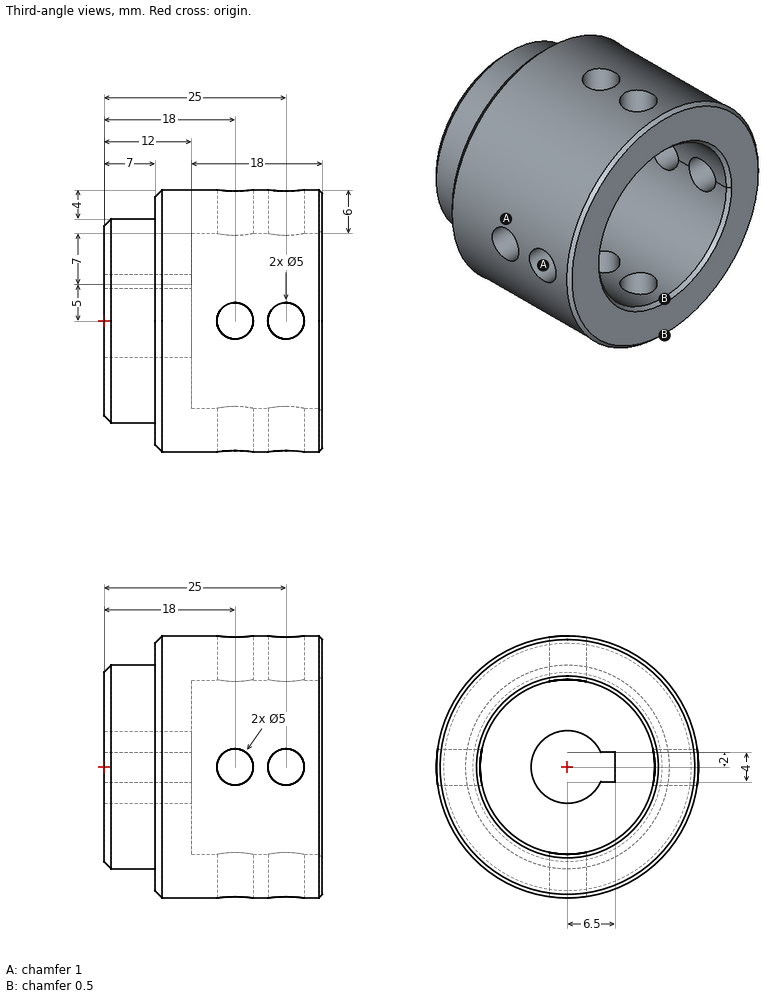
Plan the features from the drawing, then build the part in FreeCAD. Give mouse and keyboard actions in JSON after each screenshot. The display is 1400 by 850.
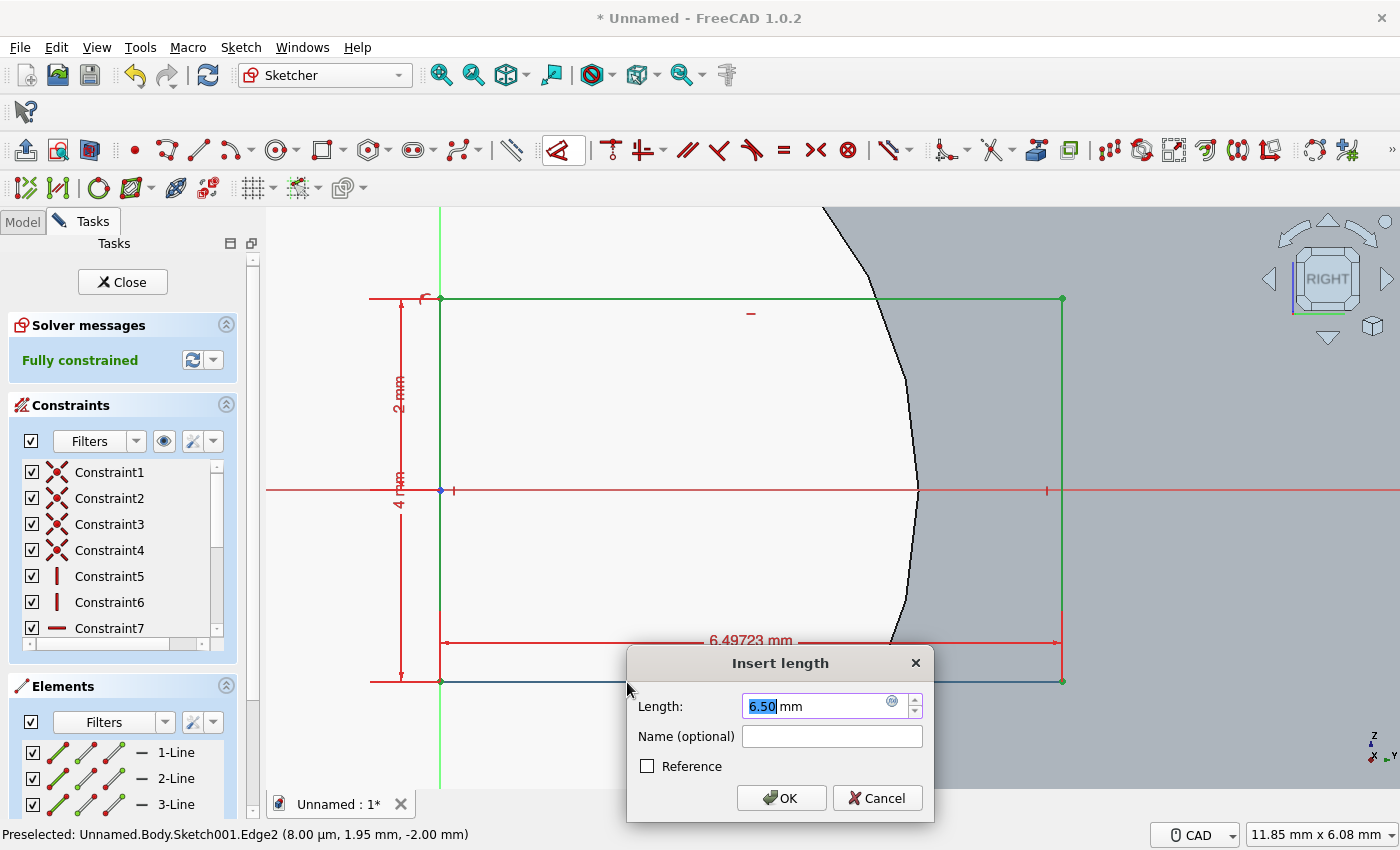
{"action": "type", "text": "6.5"}
{"action": "key", "text": "Return"}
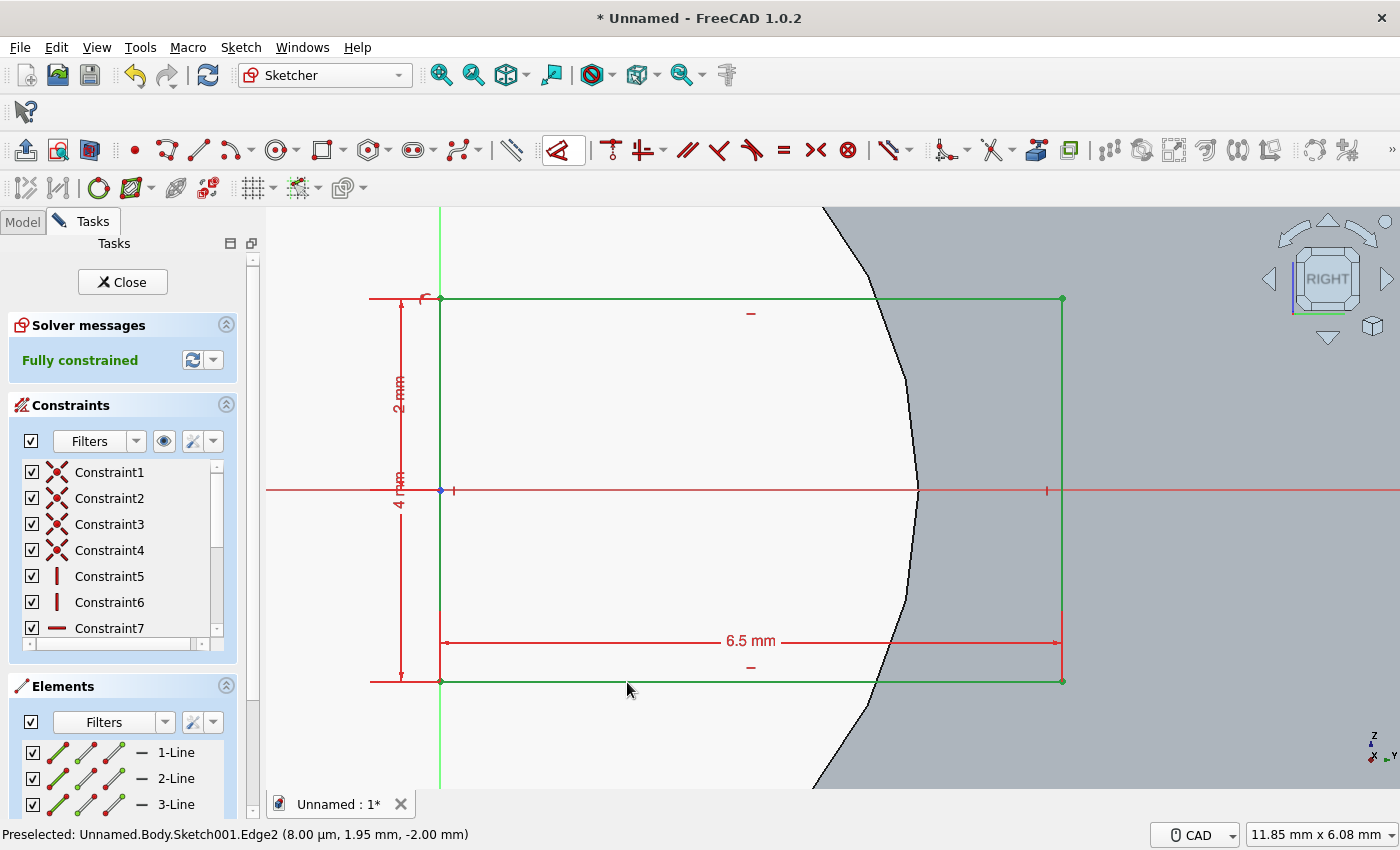
{"action": "left_click", "coordinate": [123, 282]}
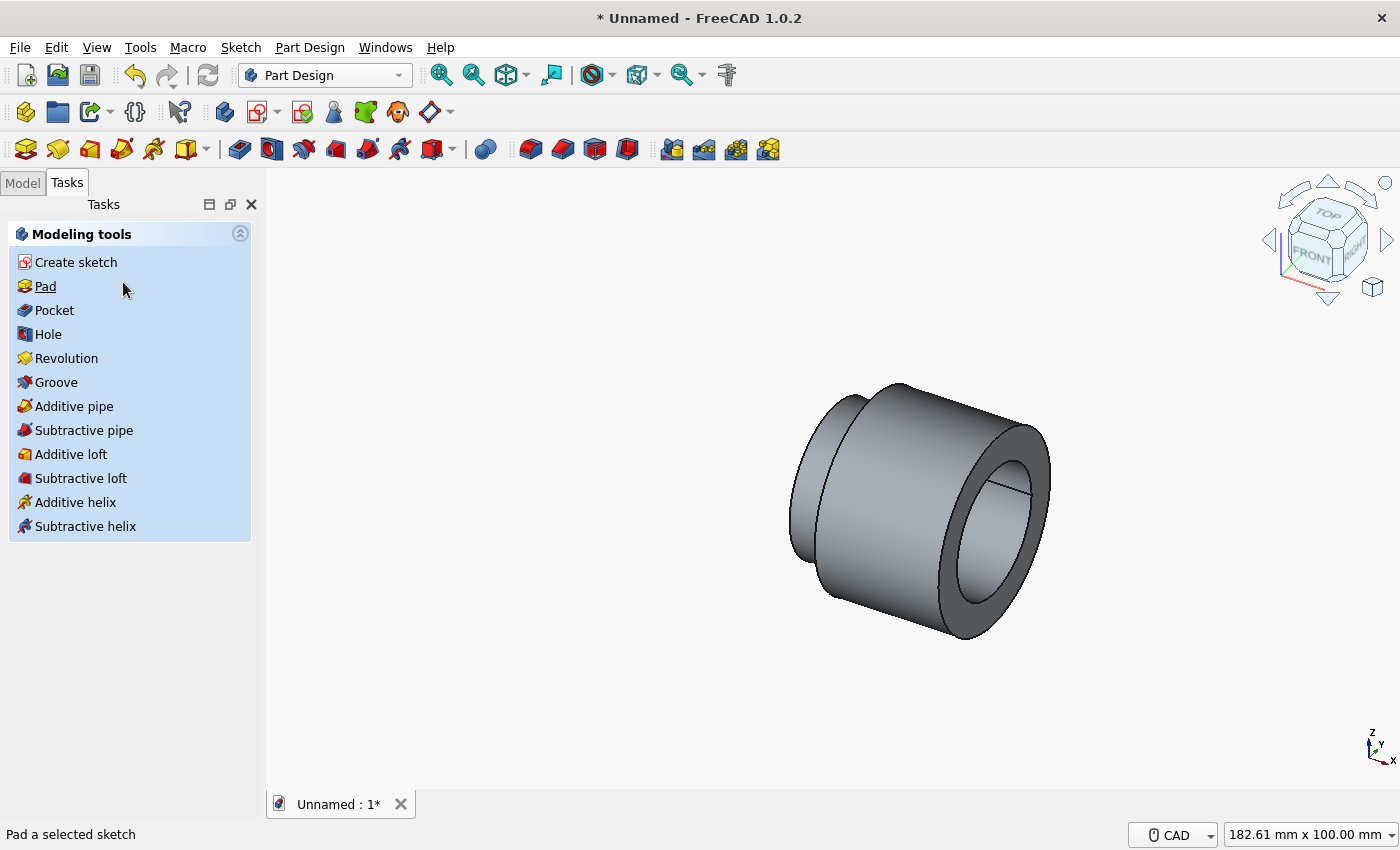
{"action": "left_click", "coordinate": [240, 150]}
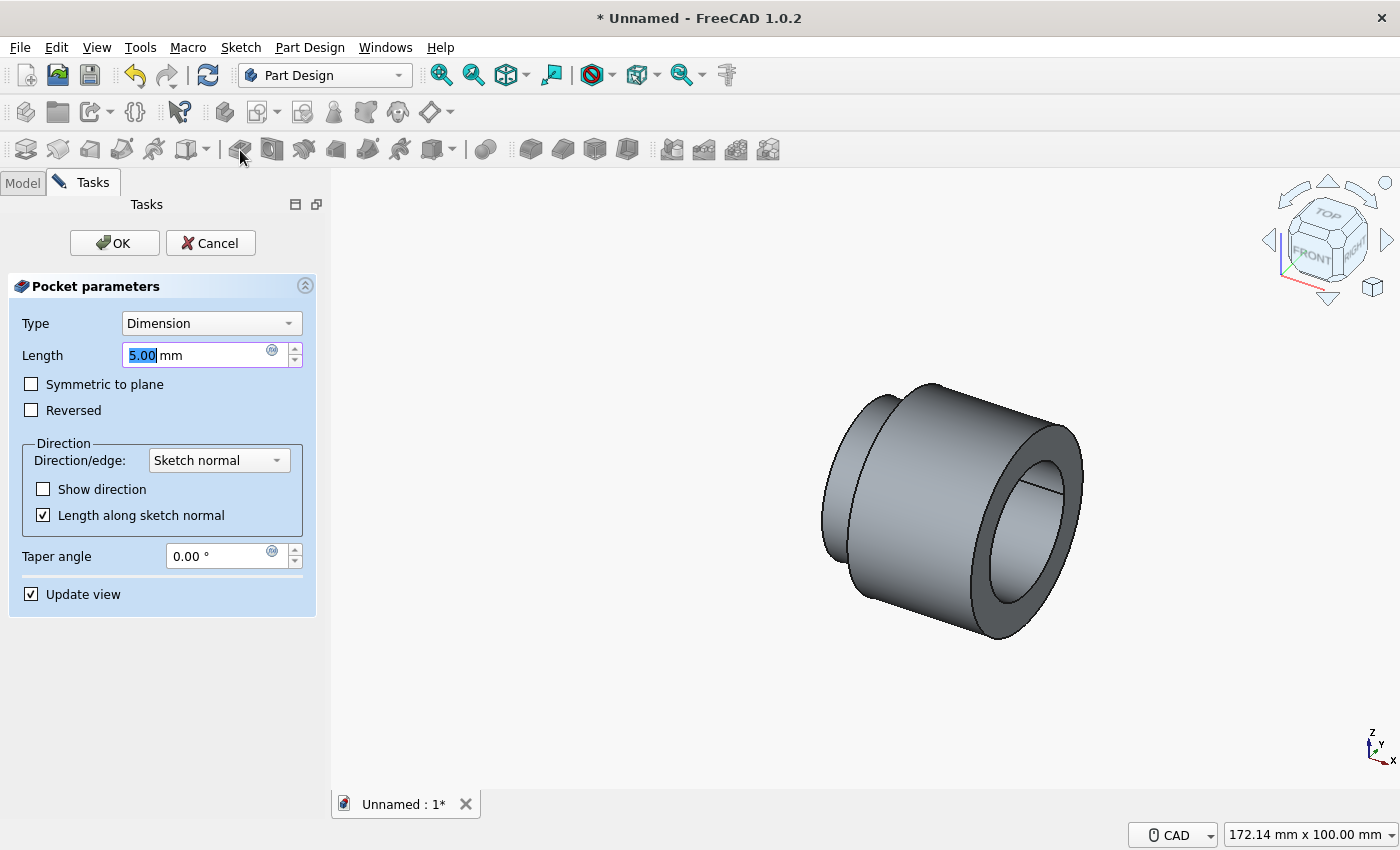
{"action": "left_click", "coordinate": [212, 324]}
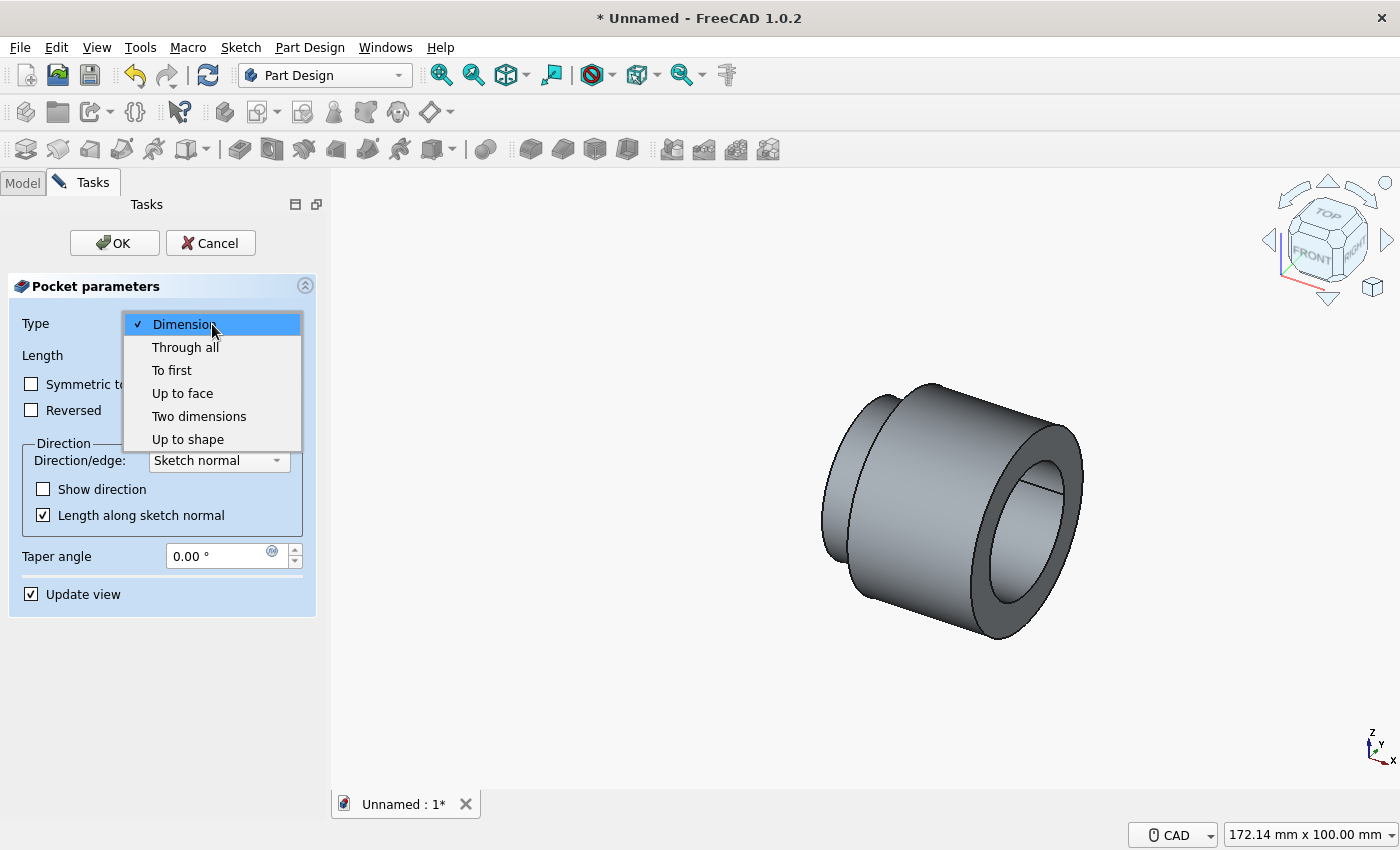
{"action": "left_click", "coordinate": [212, 348]}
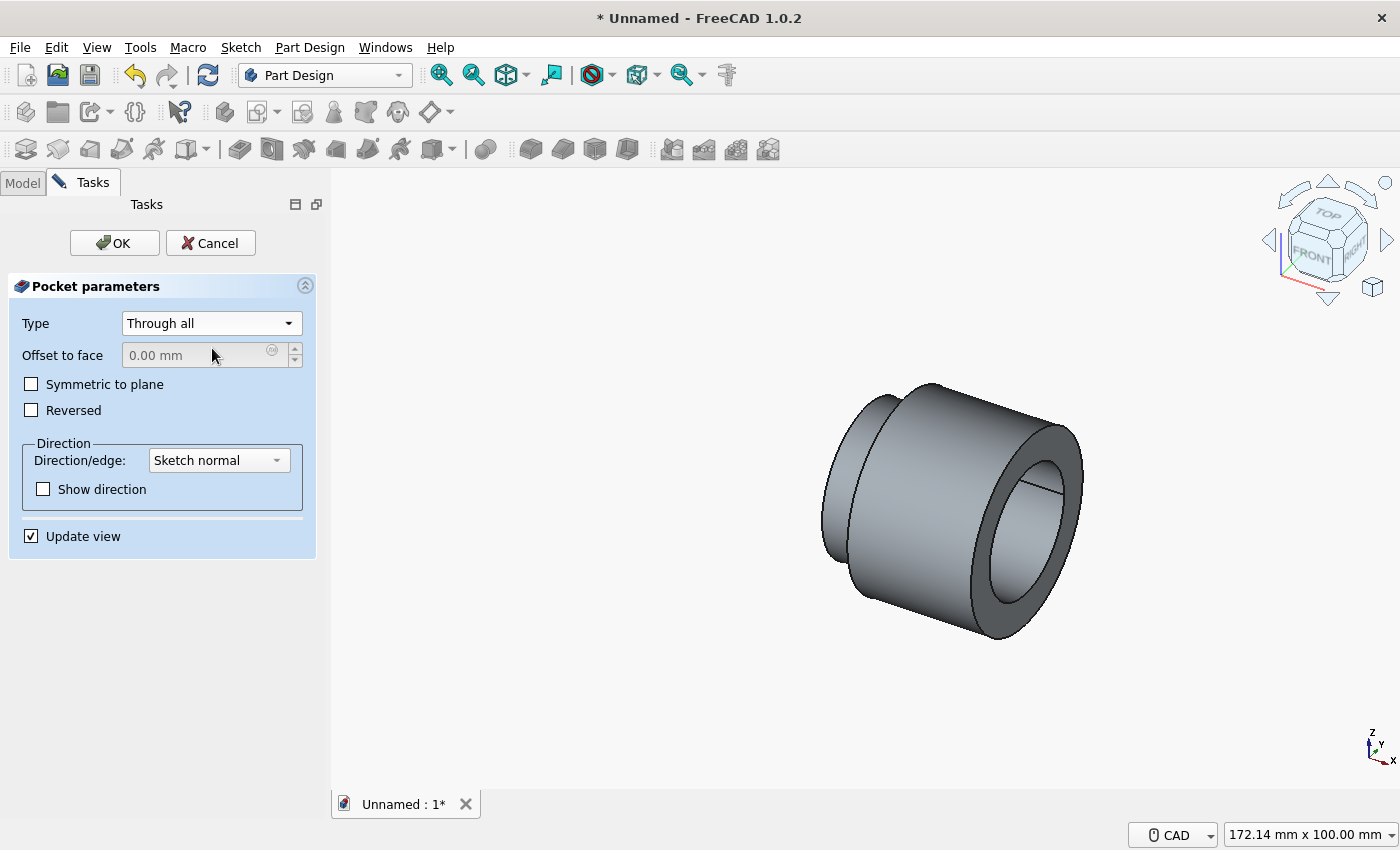
{"action": "left_click", "coordinate": [30, 410]}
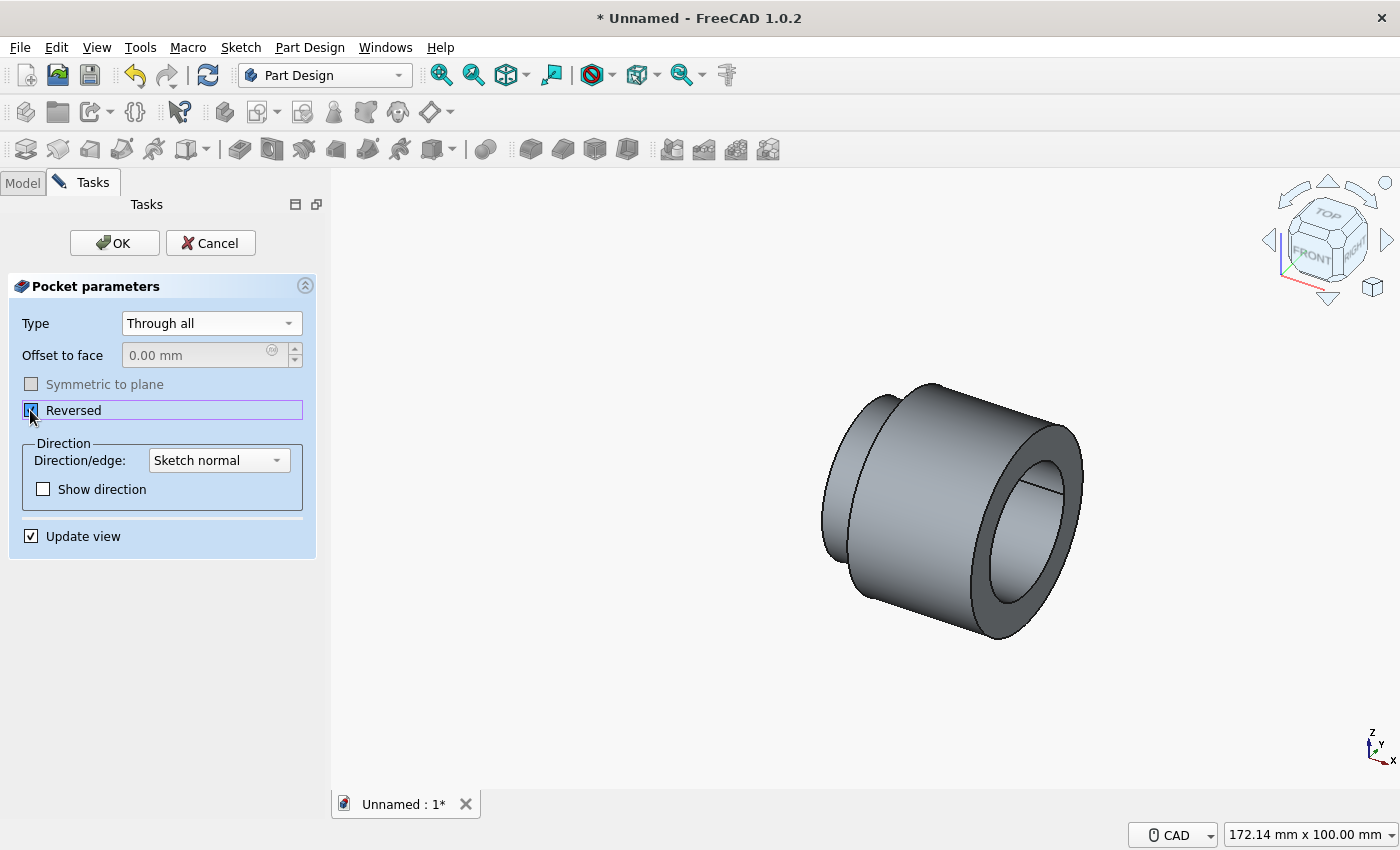
{"action": "left_click", "coordinate": [115, 243]}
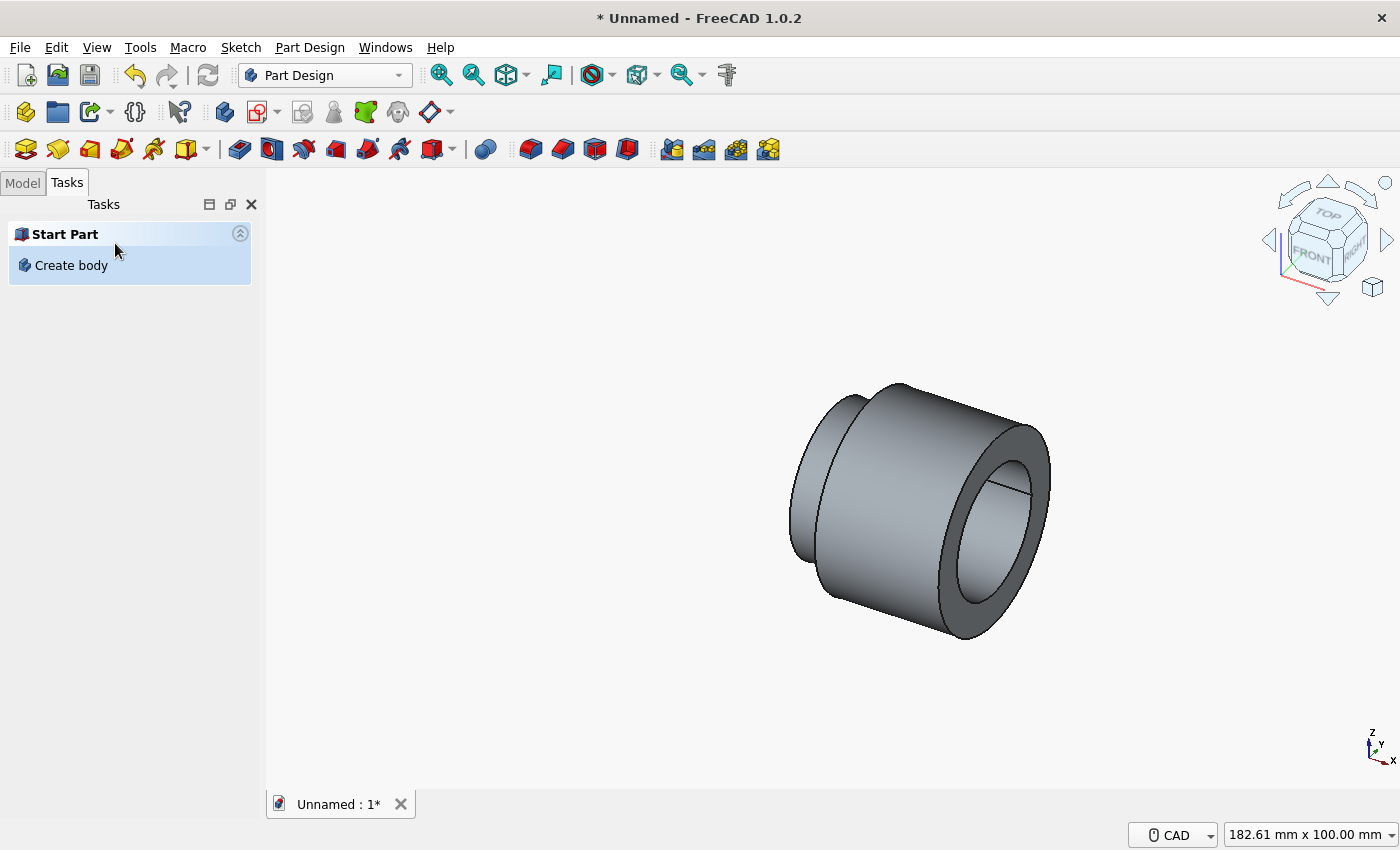
{"action": "left_click", "coordinate": [258, 112]}